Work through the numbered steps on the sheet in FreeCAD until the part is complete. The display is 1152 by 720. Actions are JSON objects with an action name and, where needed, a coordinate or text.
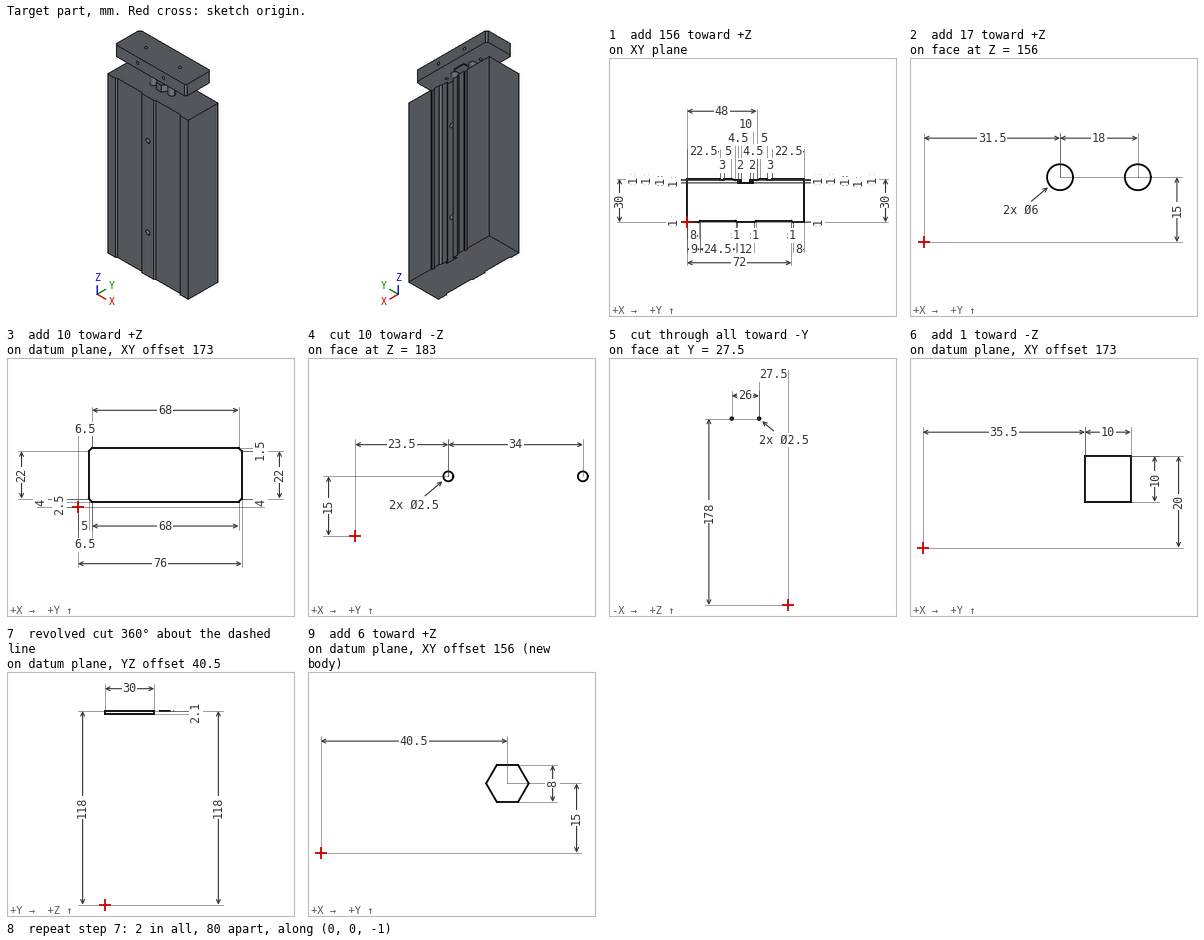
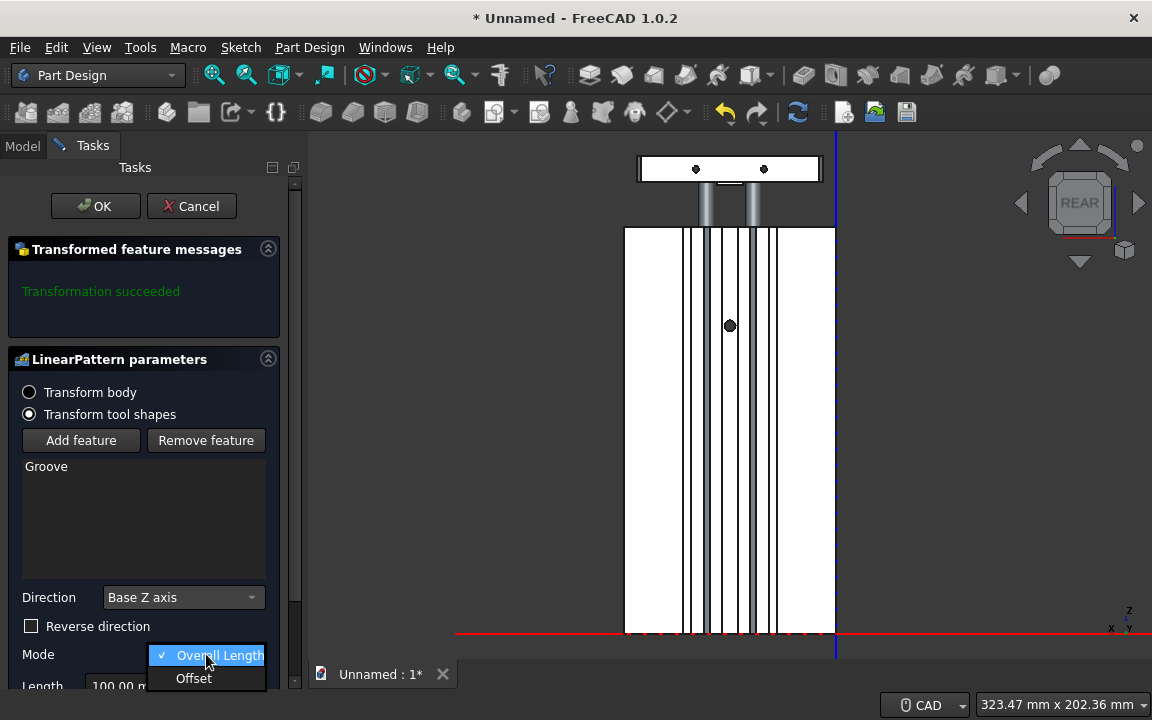
{"action": "left_click", "coordinate": [206, 678]}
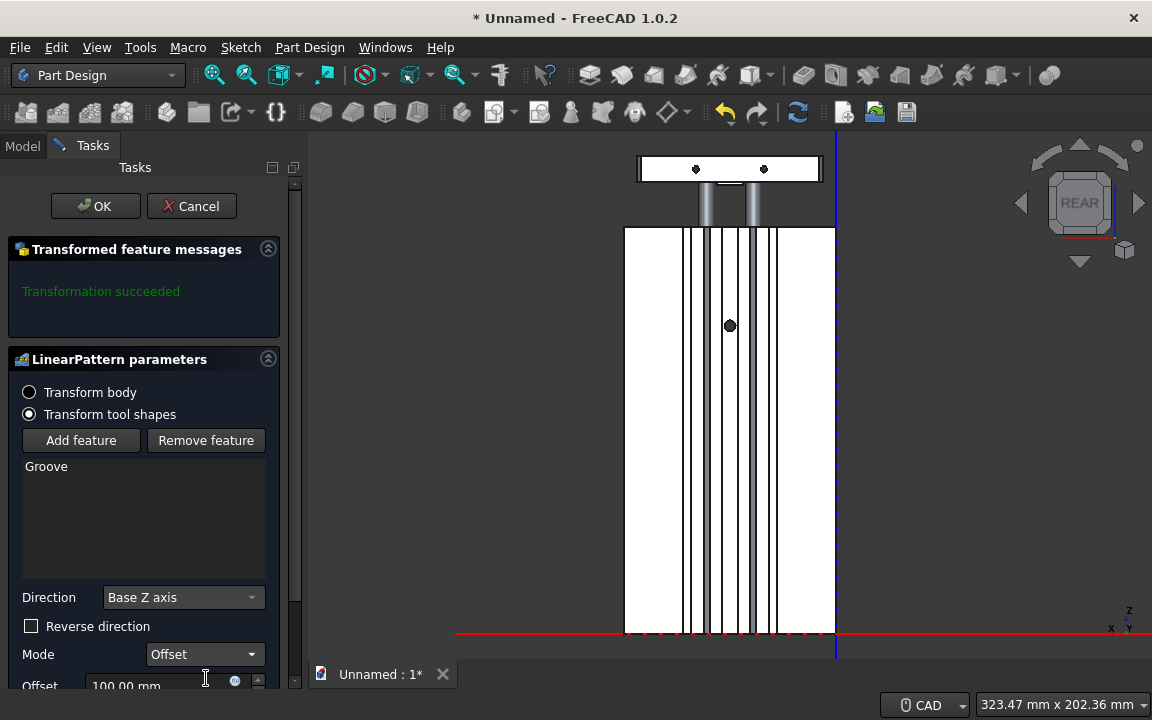
{"action": "scroll", "coordinate": [295, 432], "scroll_direction": "down", "scroll_amount": 2}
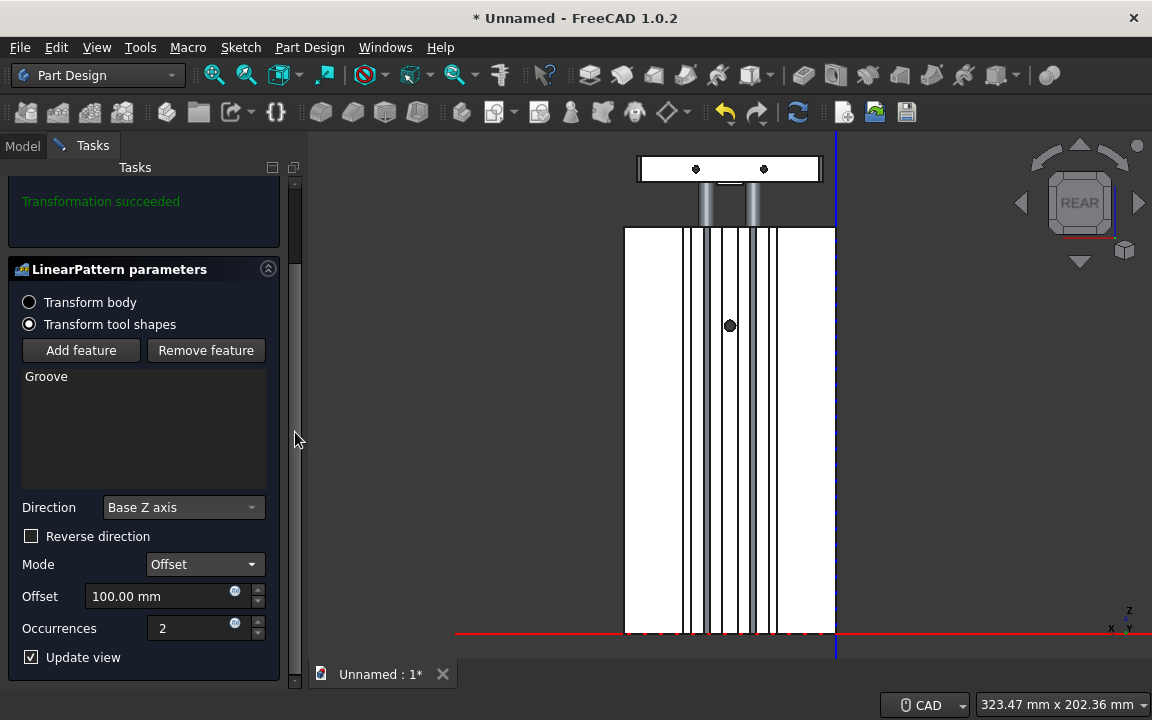
{"action": "triple_click", "coordinate": [168, 596]}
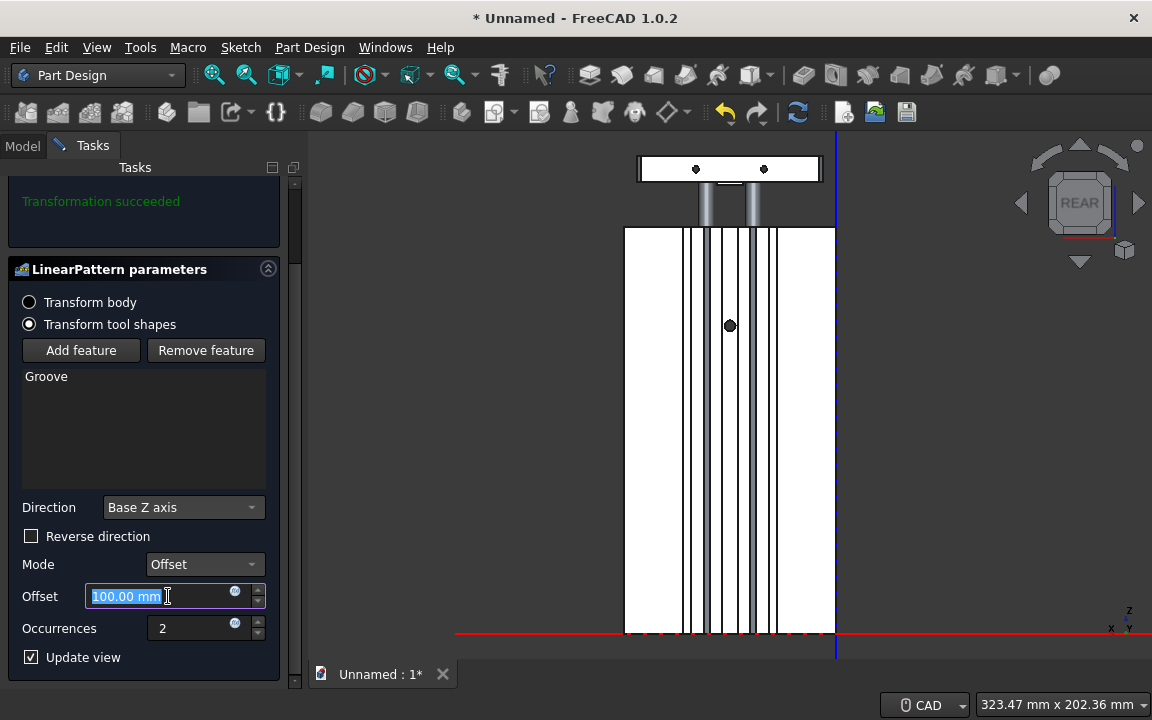
{"action": "type", "text": "80"}
{"action": "key", "text": "Tab"}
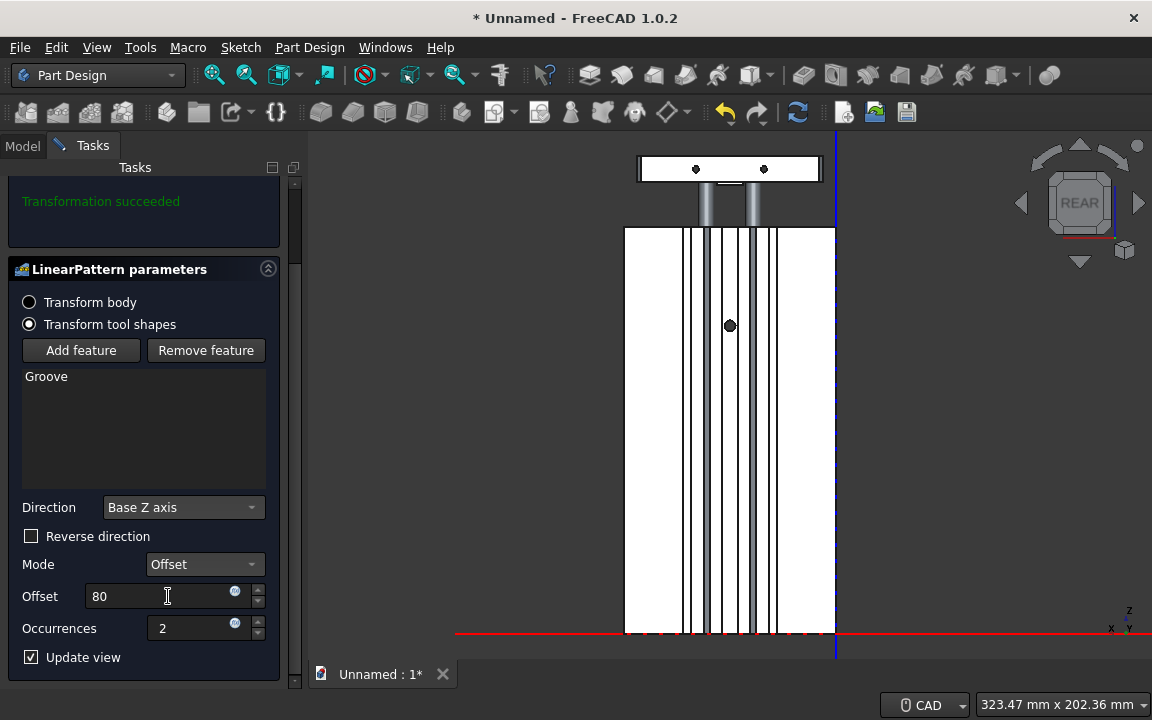
{"action": "triple_click", "coordinate": [198, 628]}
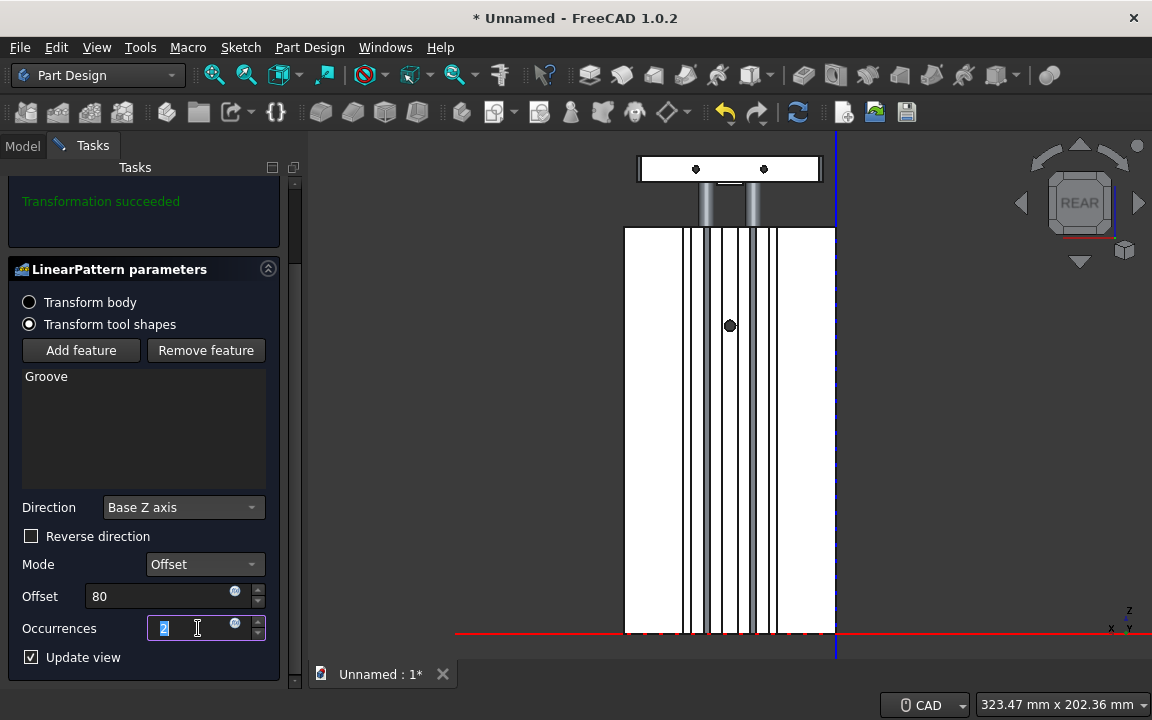
{"action": "type", "text": "2"}
{"action": "key", "text": "Tab"}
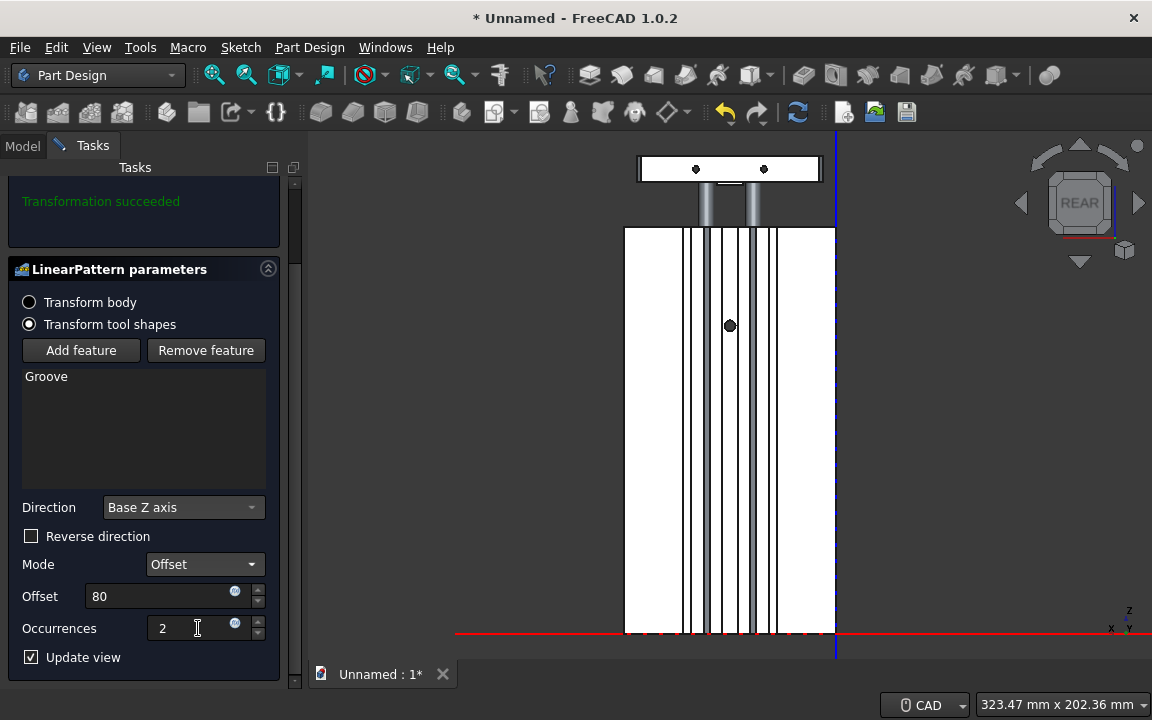
{"action": "left_click", "coordinate": [30, 536]}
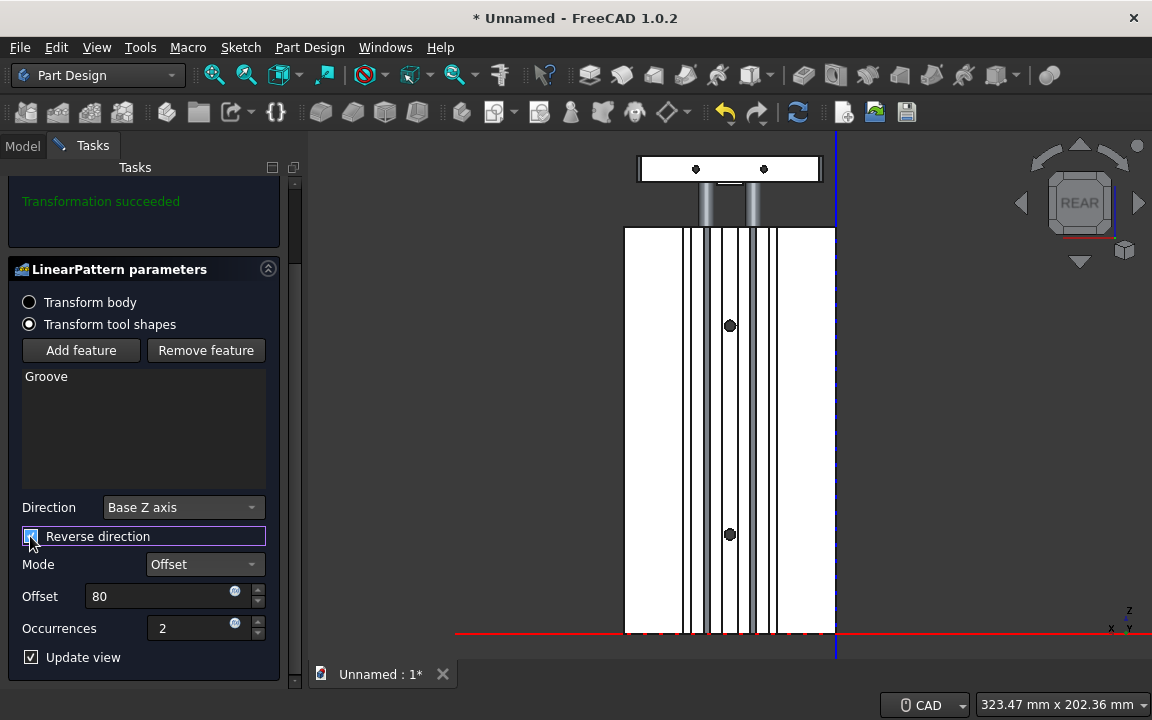
{"action": "scroll", "coordinate": [295, 432], "scroll_direction": "up", "scroll_amount": 3}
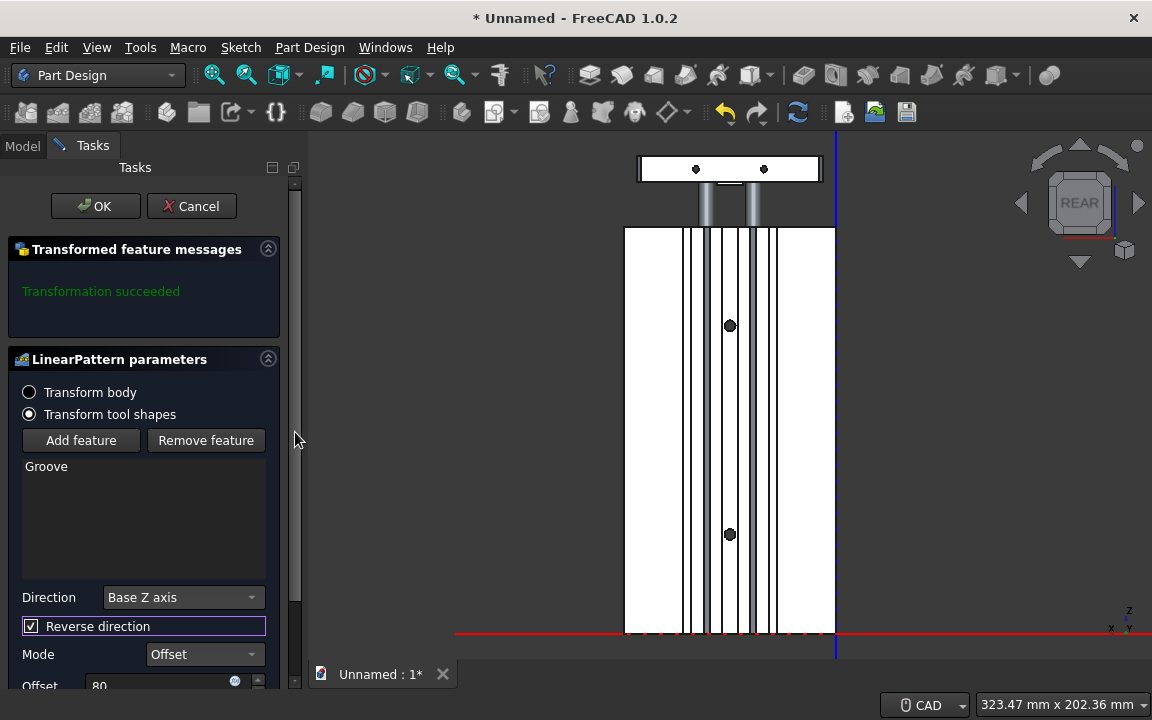
{"action": "left_click", "coordinate": [96, 206]}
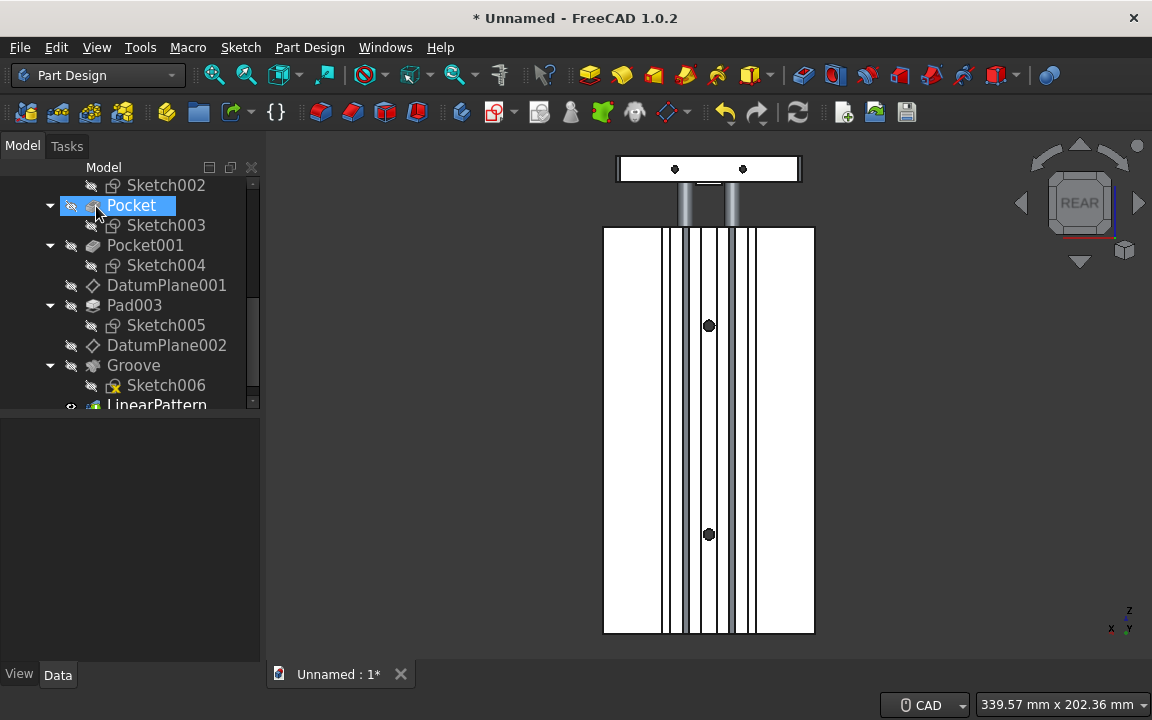
{"action": "left_click", "coordinate": [462, 112]}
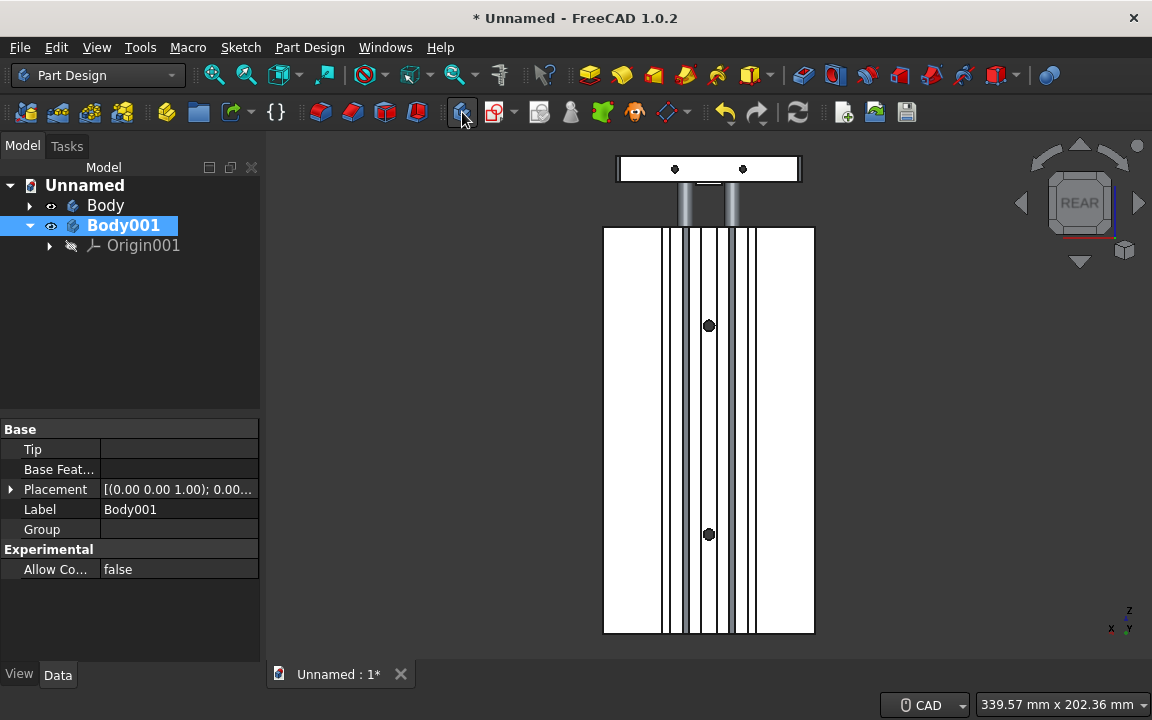
{"action": "left_click", "coordinate": [50, 246]}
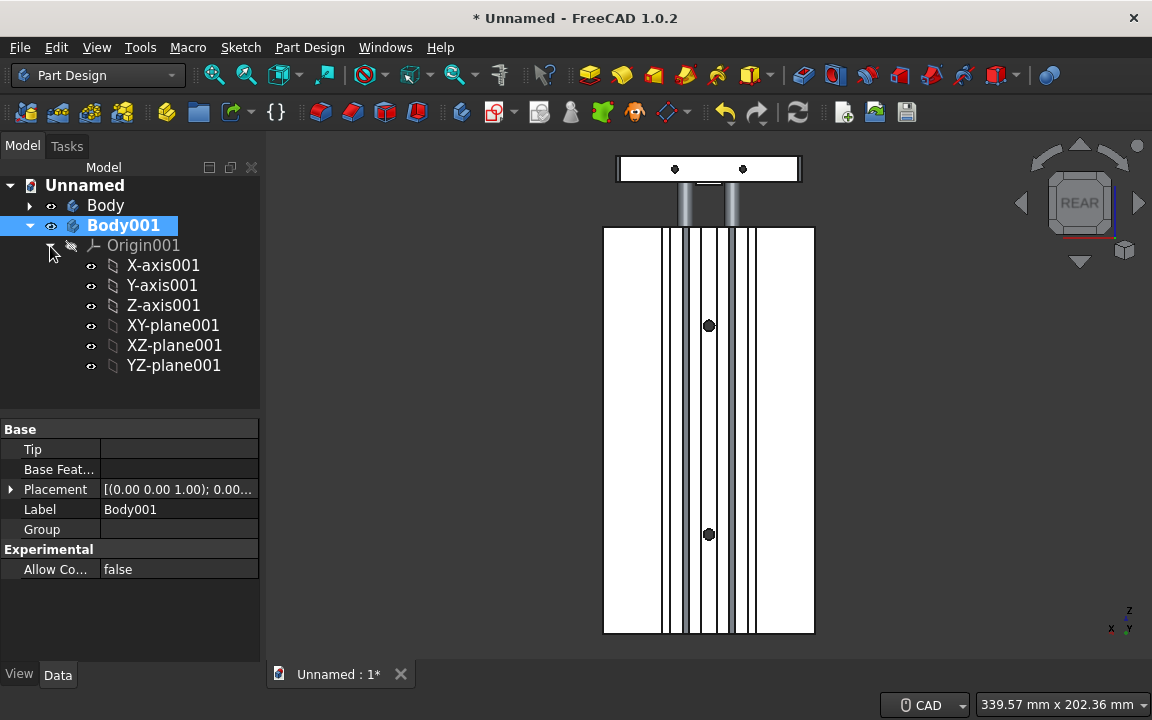
{"action": "left_click", "coordinate": [136, 326]}